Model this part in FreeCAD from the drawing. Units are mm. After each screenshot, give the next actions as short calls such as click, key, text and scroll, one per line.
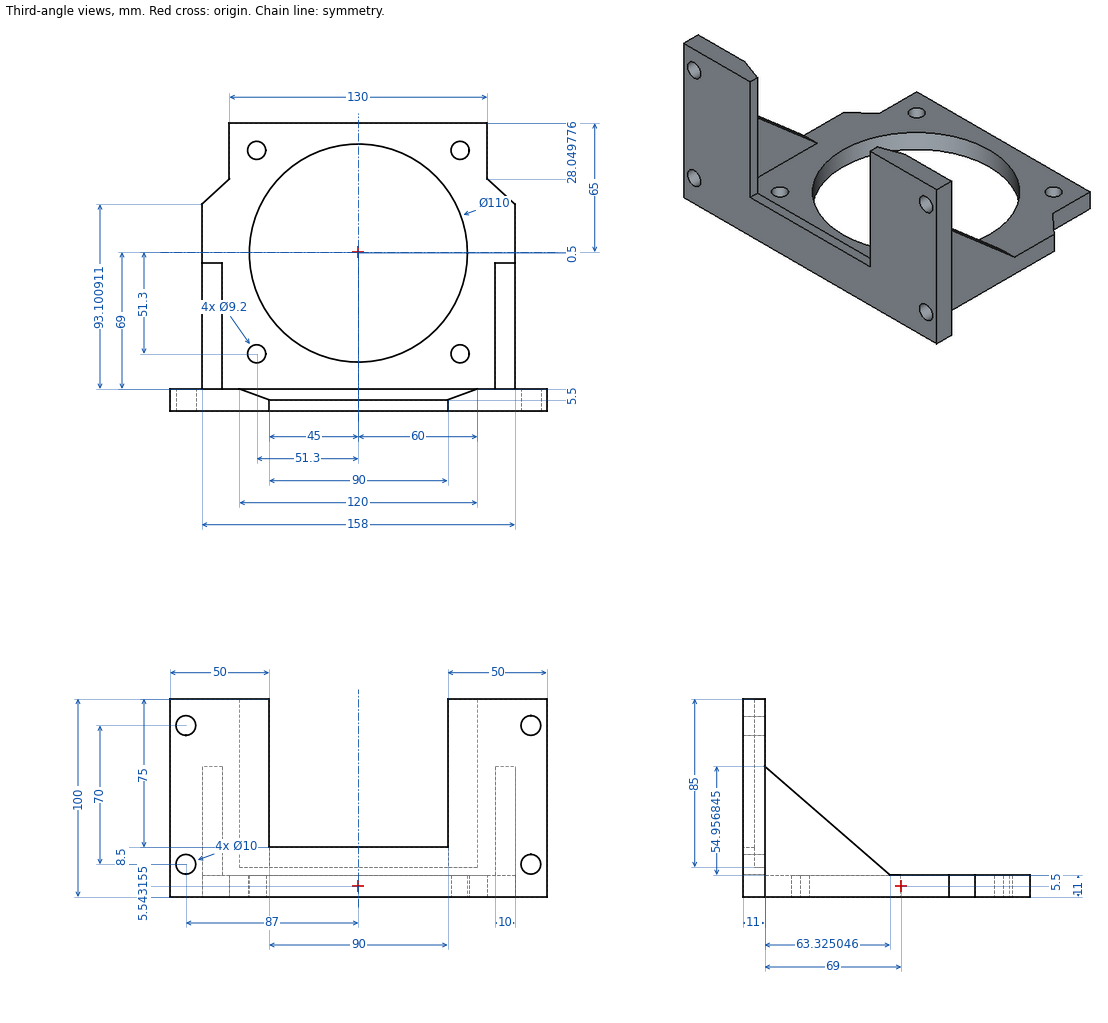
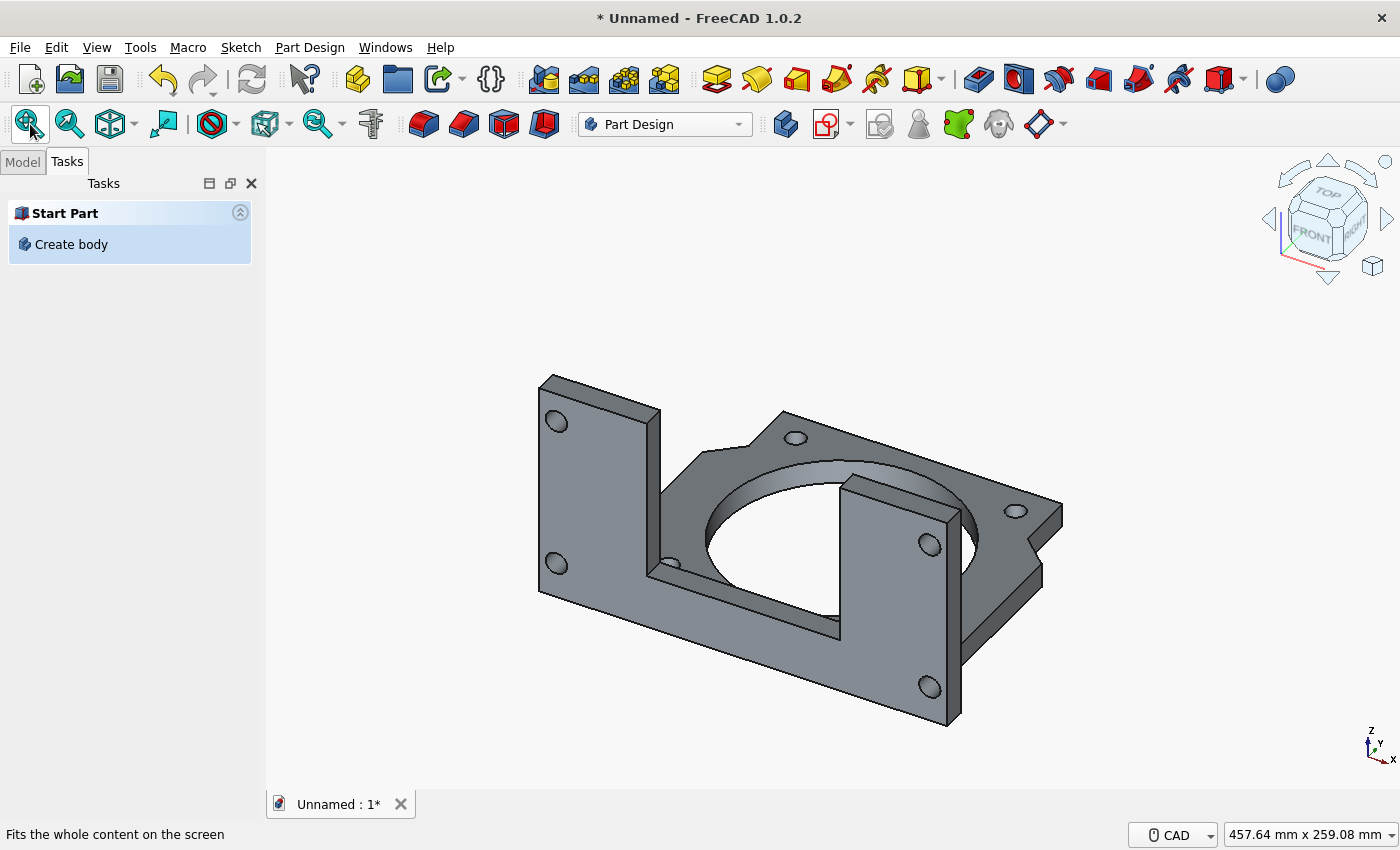
click(23, 161)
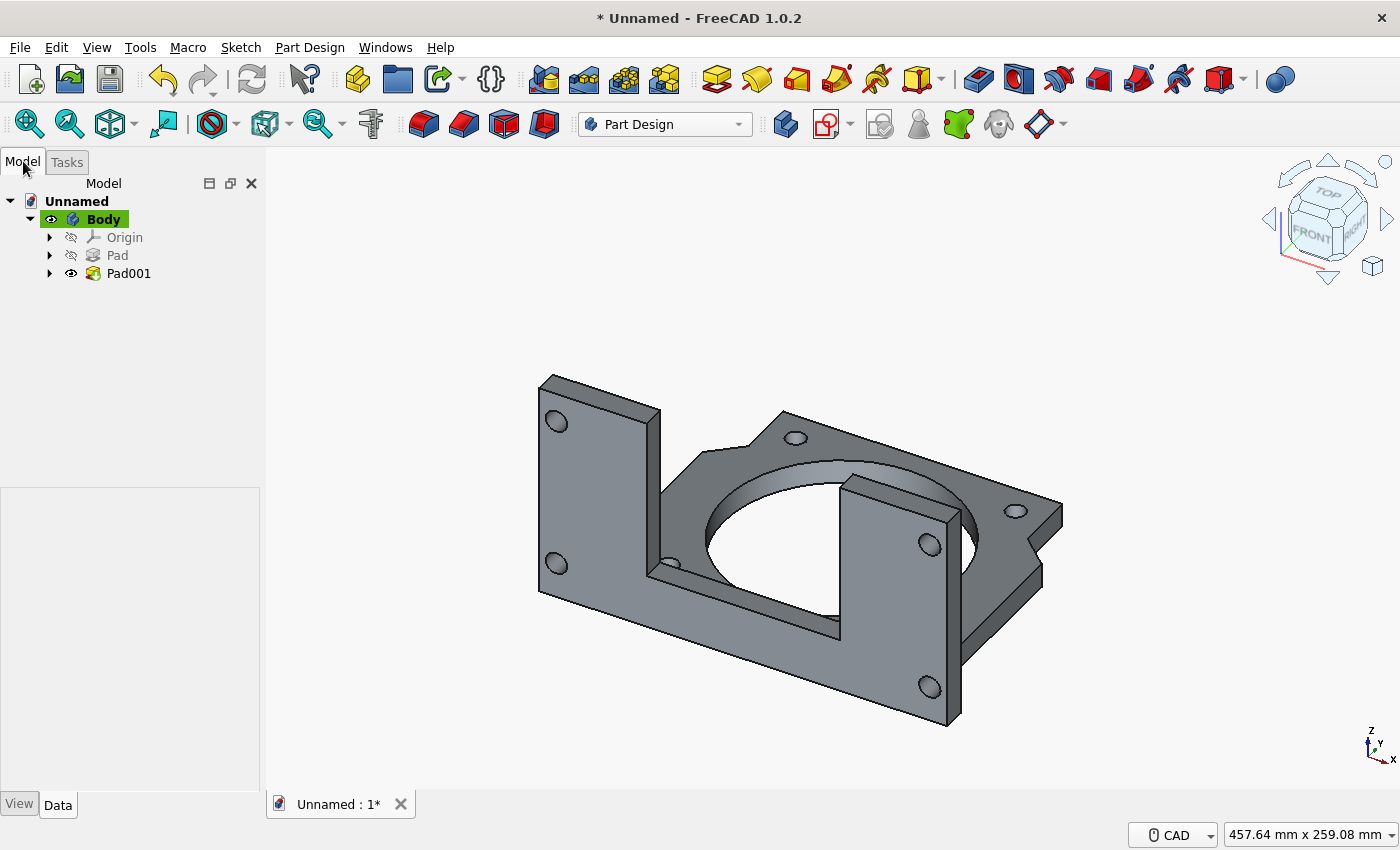
click(50, 237)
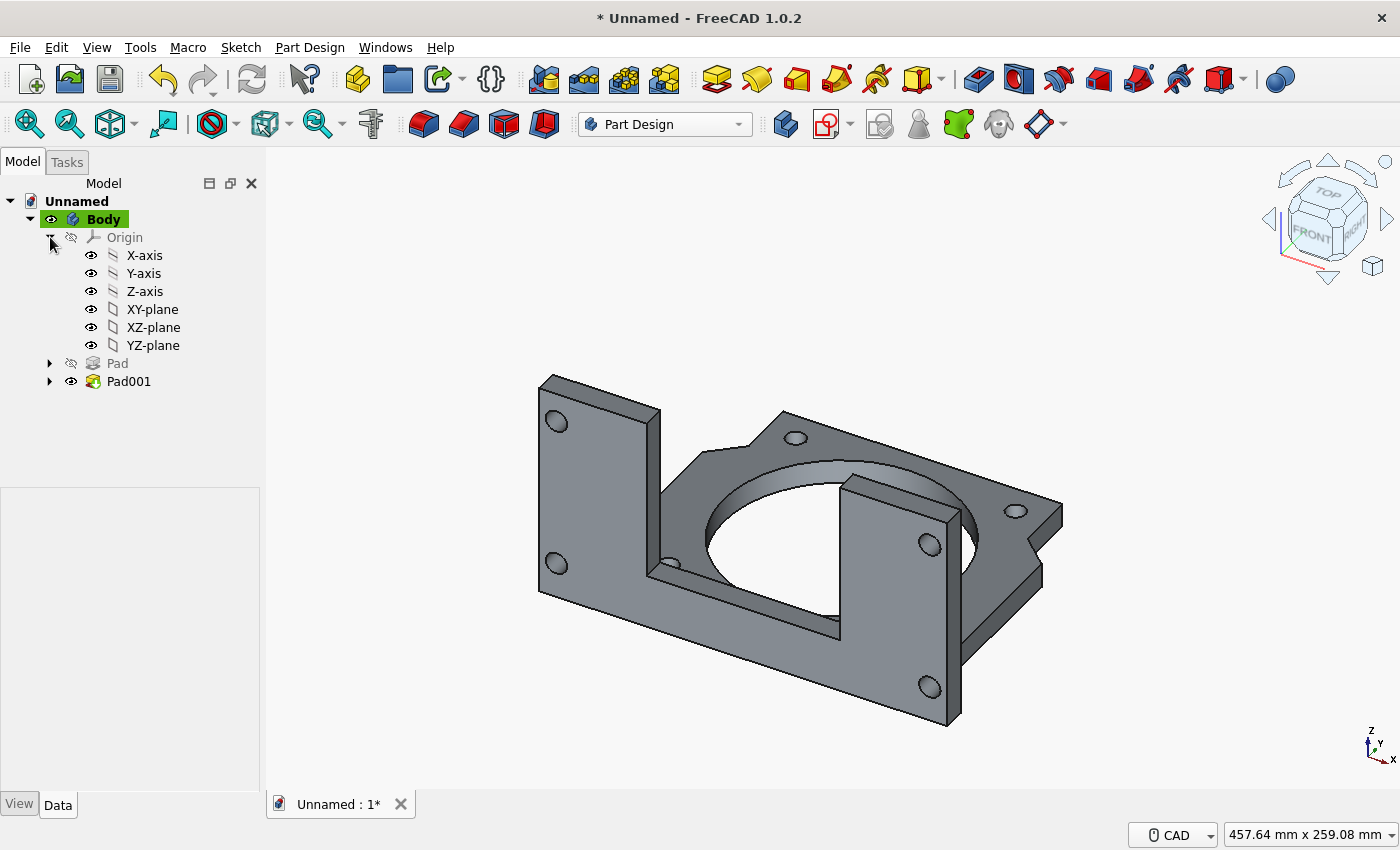
click(136, 345)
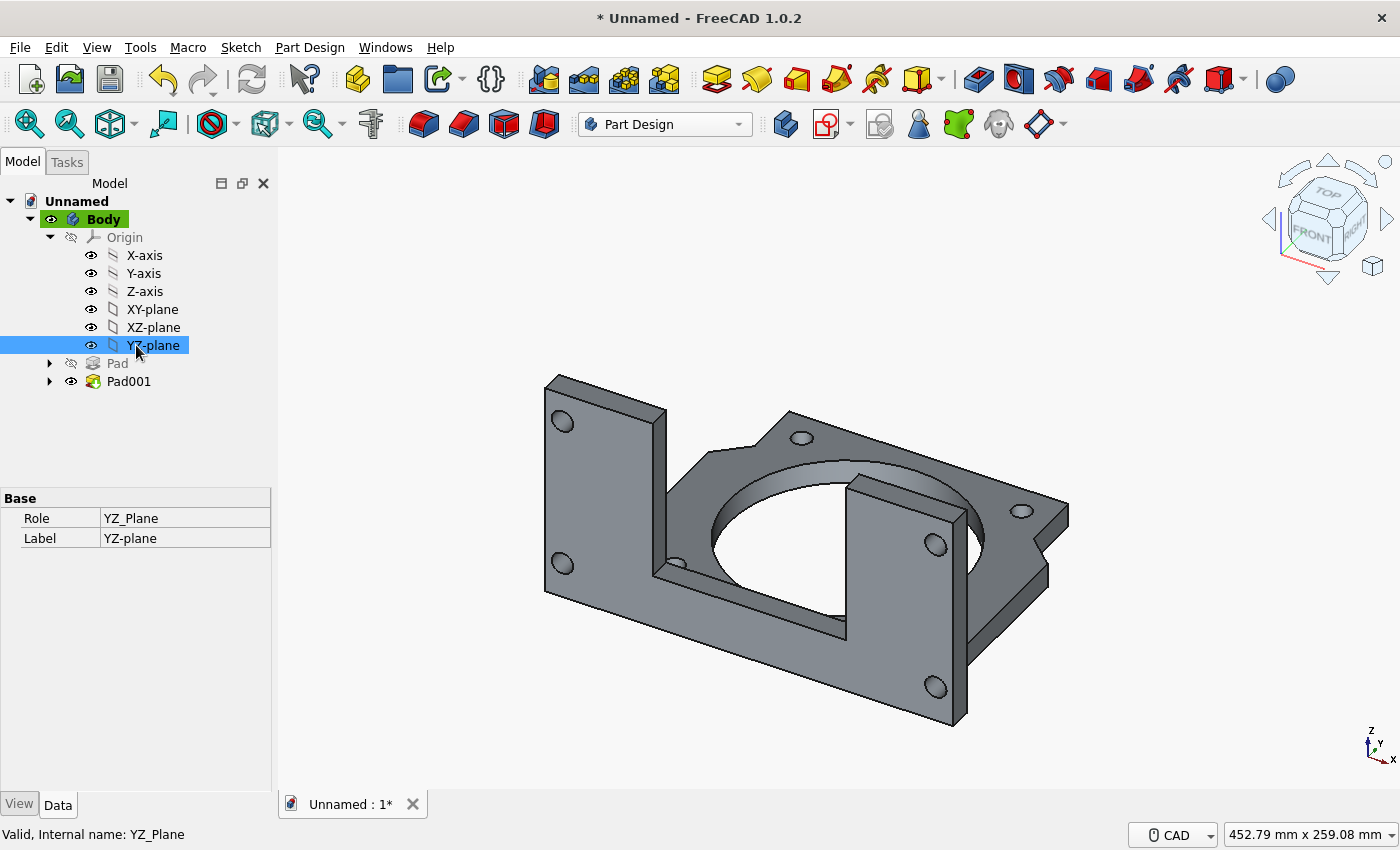
click(1040, 124)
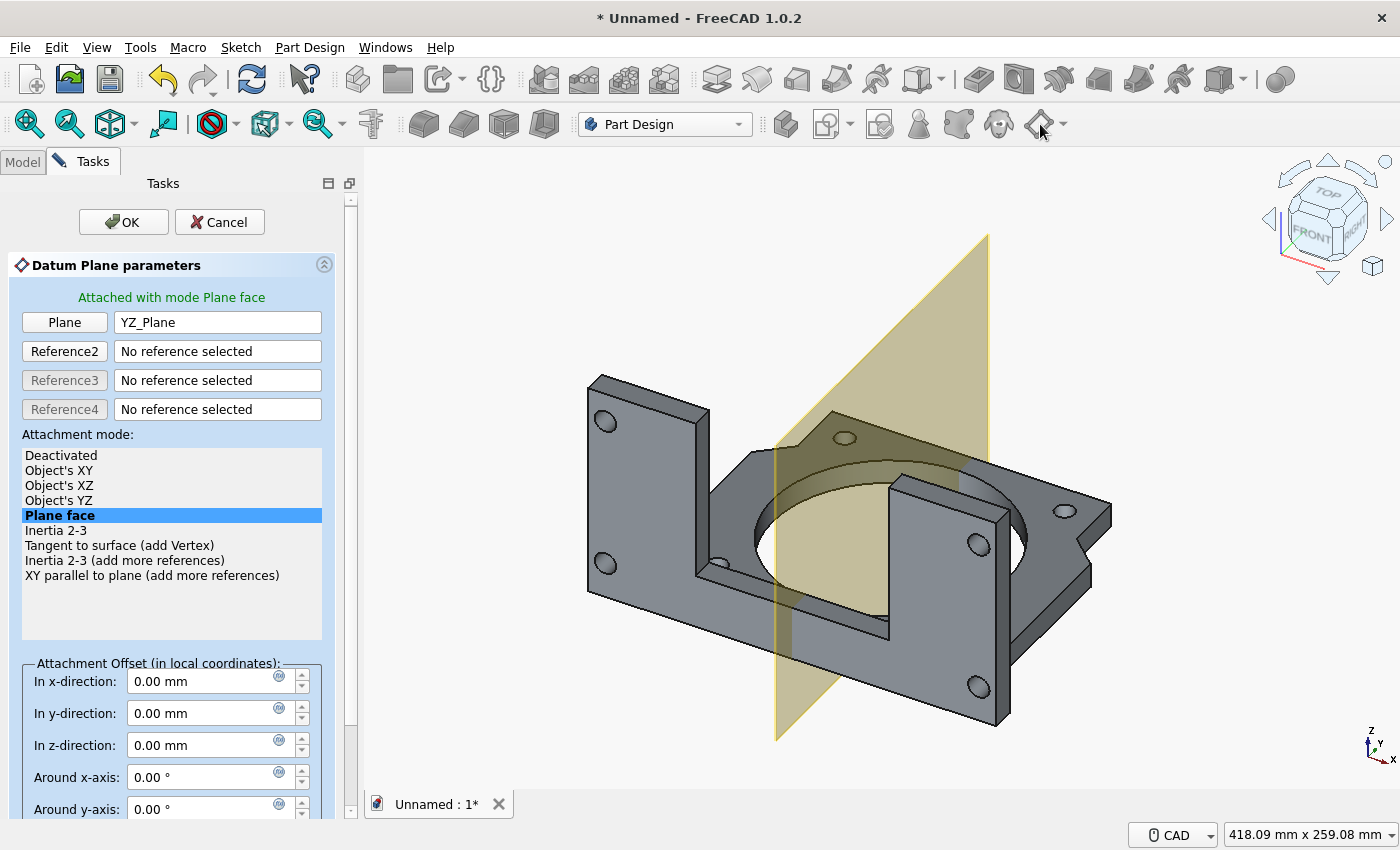
triple_click(210, 745)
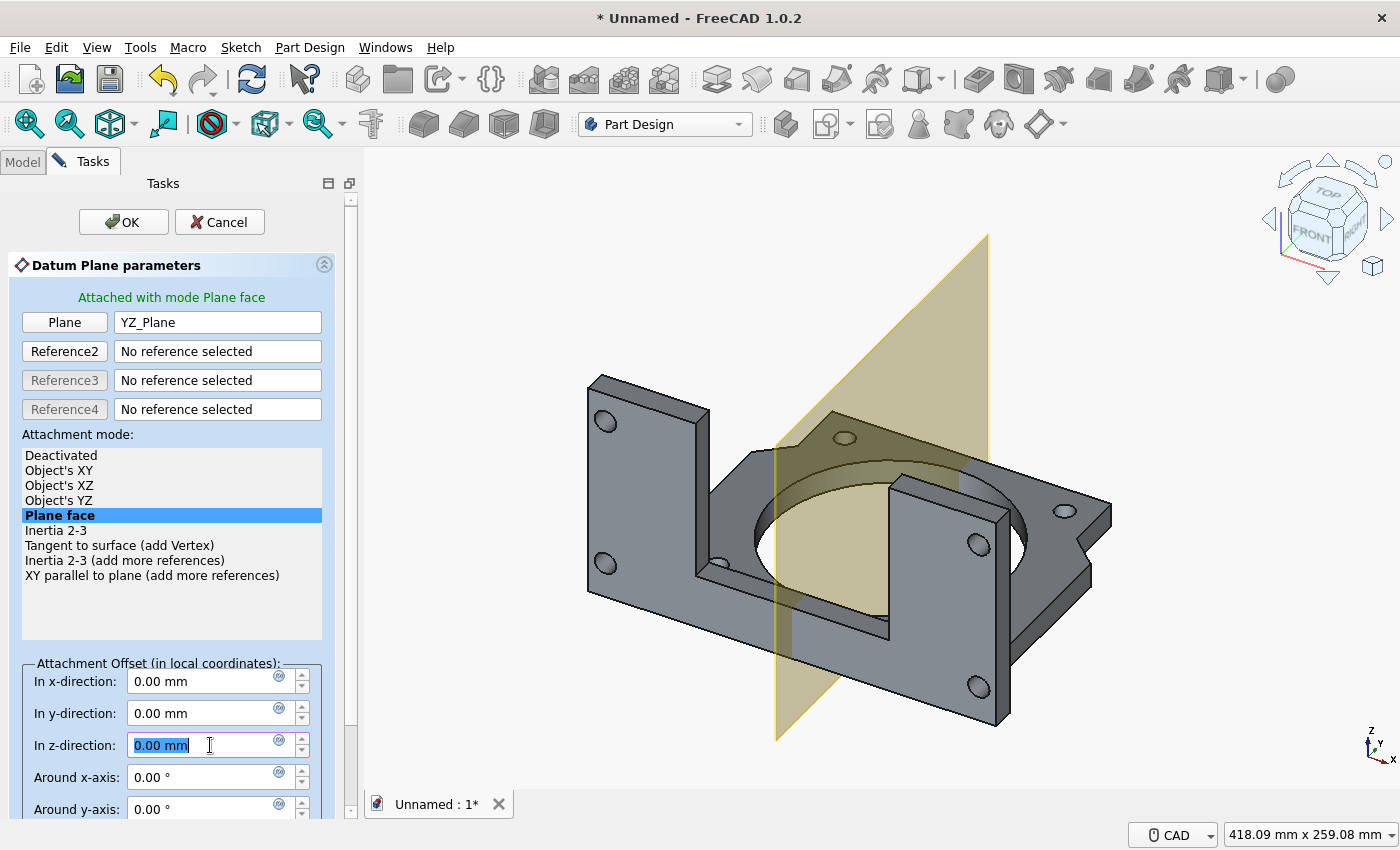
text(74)
key(Tab)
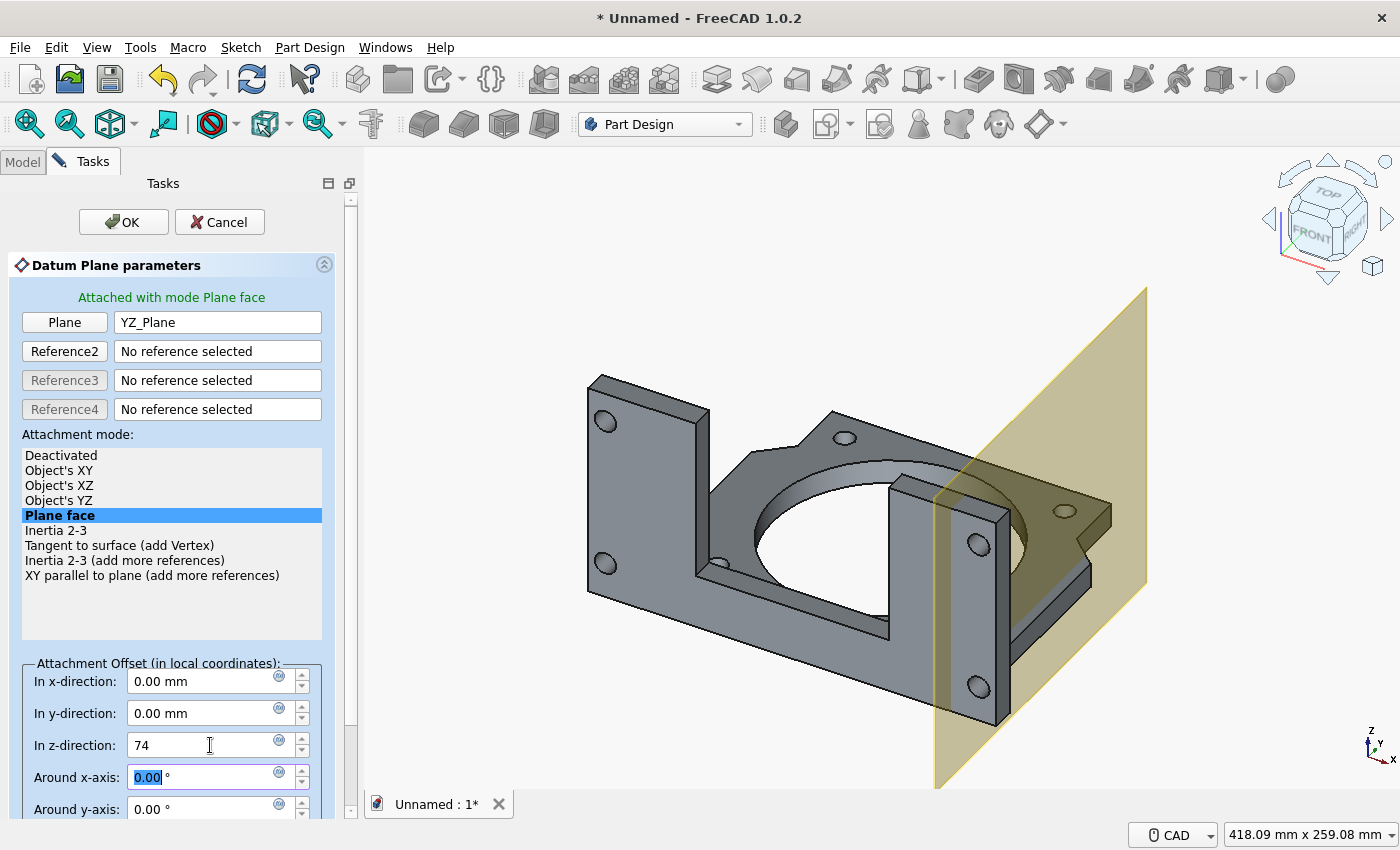
click(124, 222)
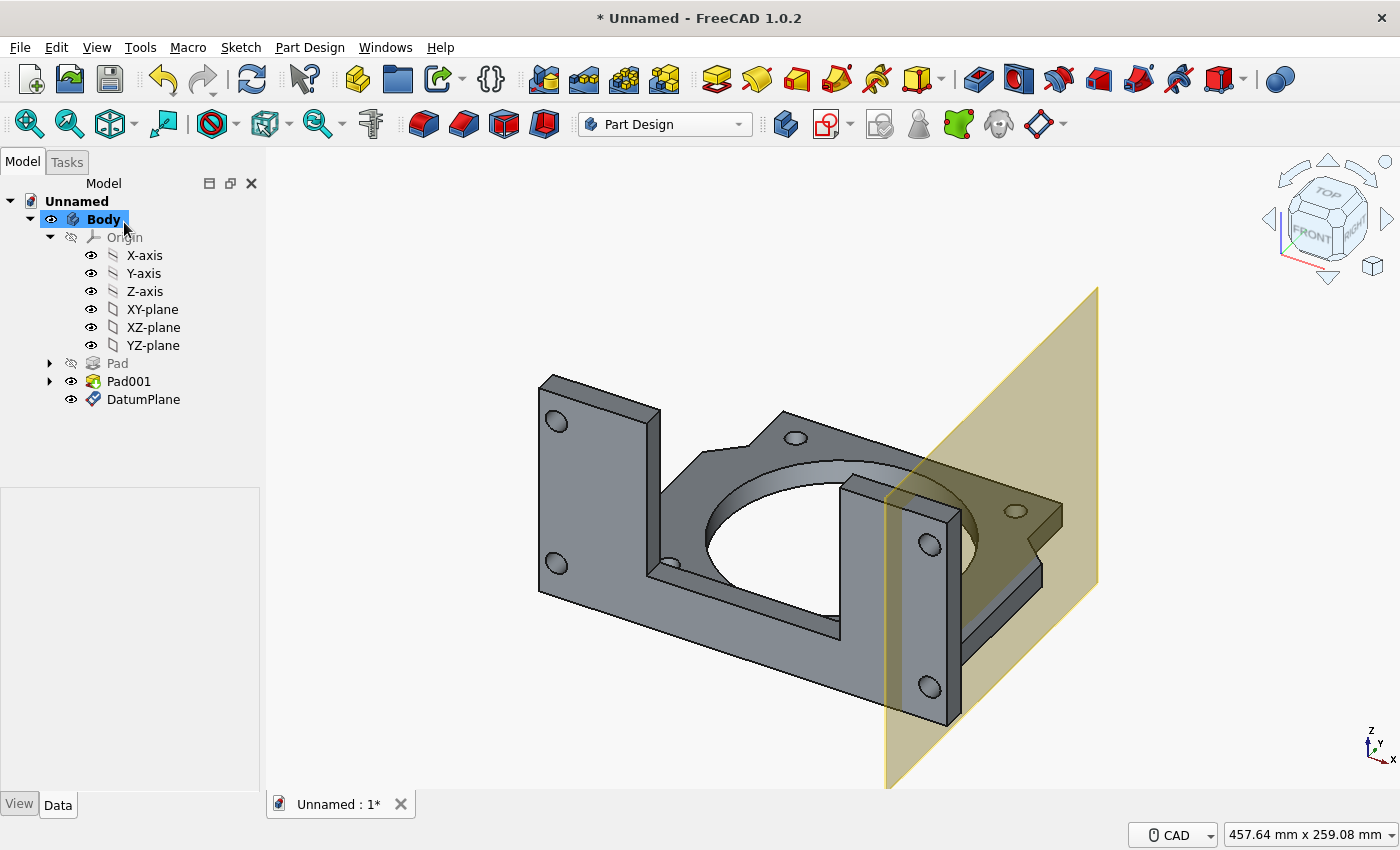
click(116, 399)